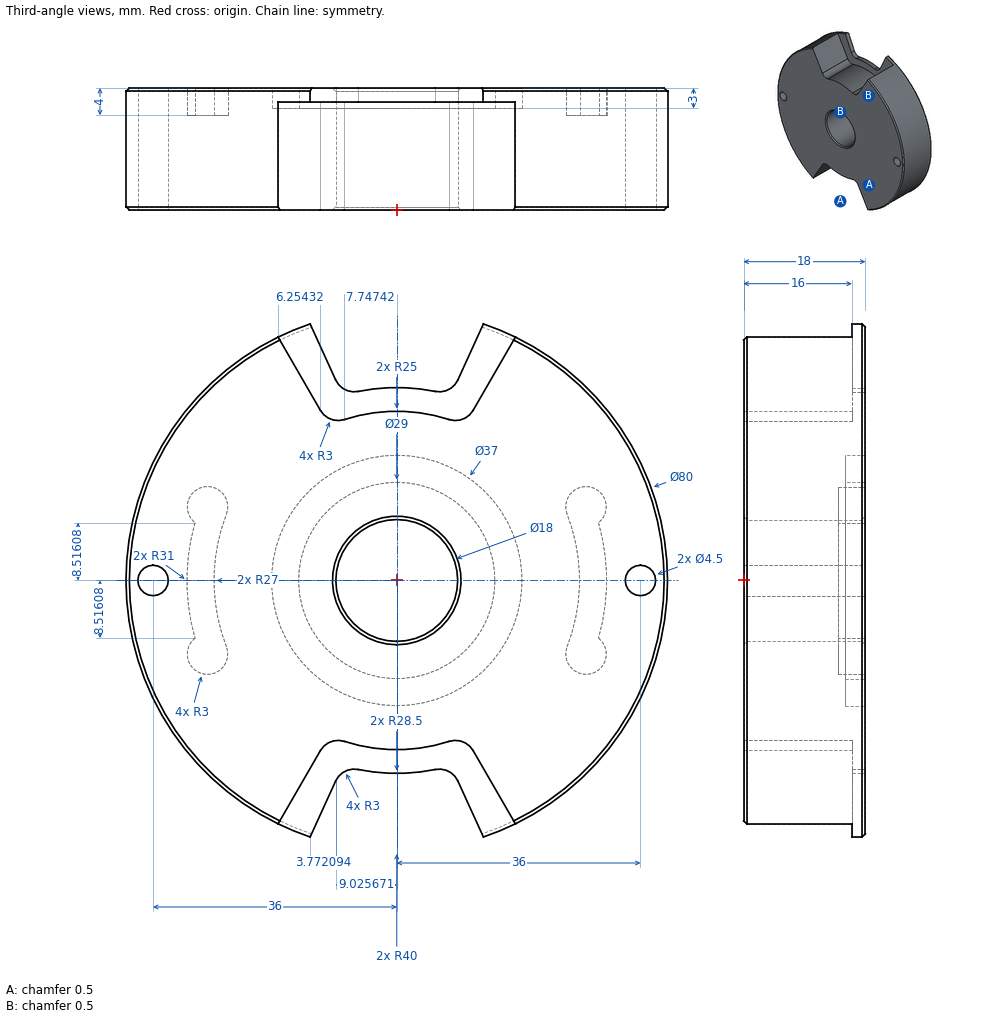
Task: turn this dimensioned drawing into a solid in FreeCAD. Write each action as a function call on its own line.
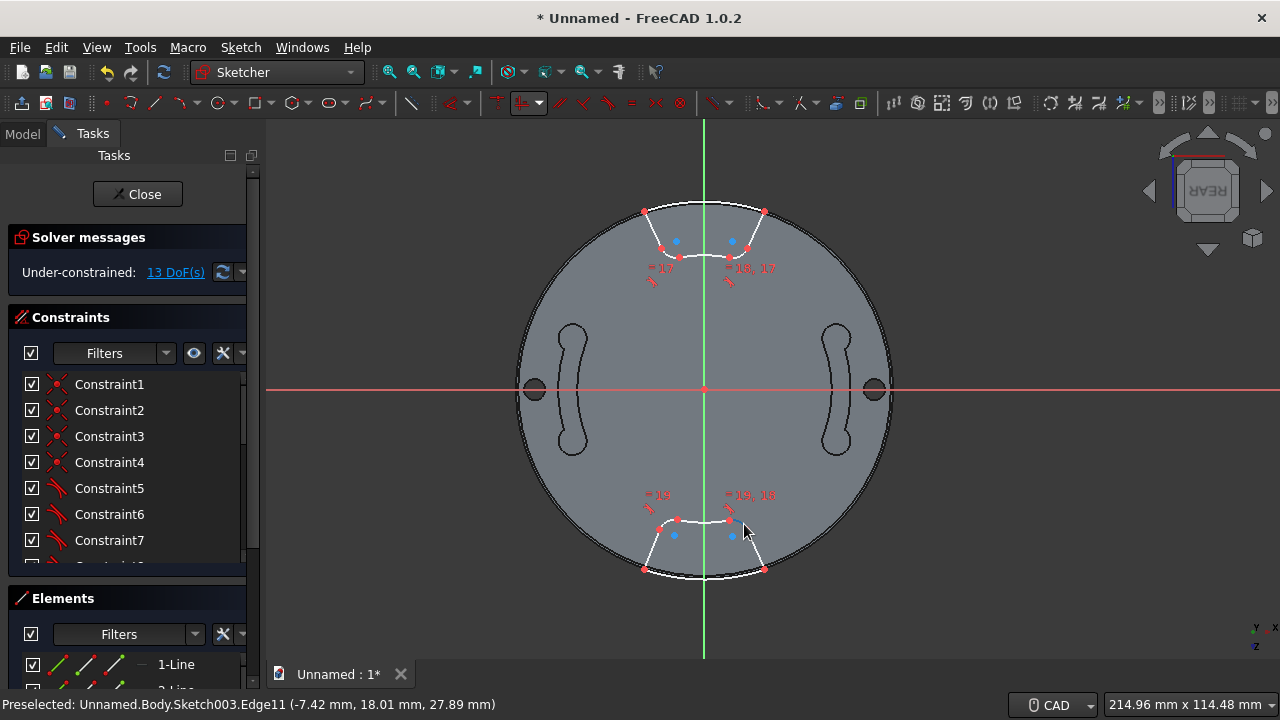
scroll(715, 256, up, 2)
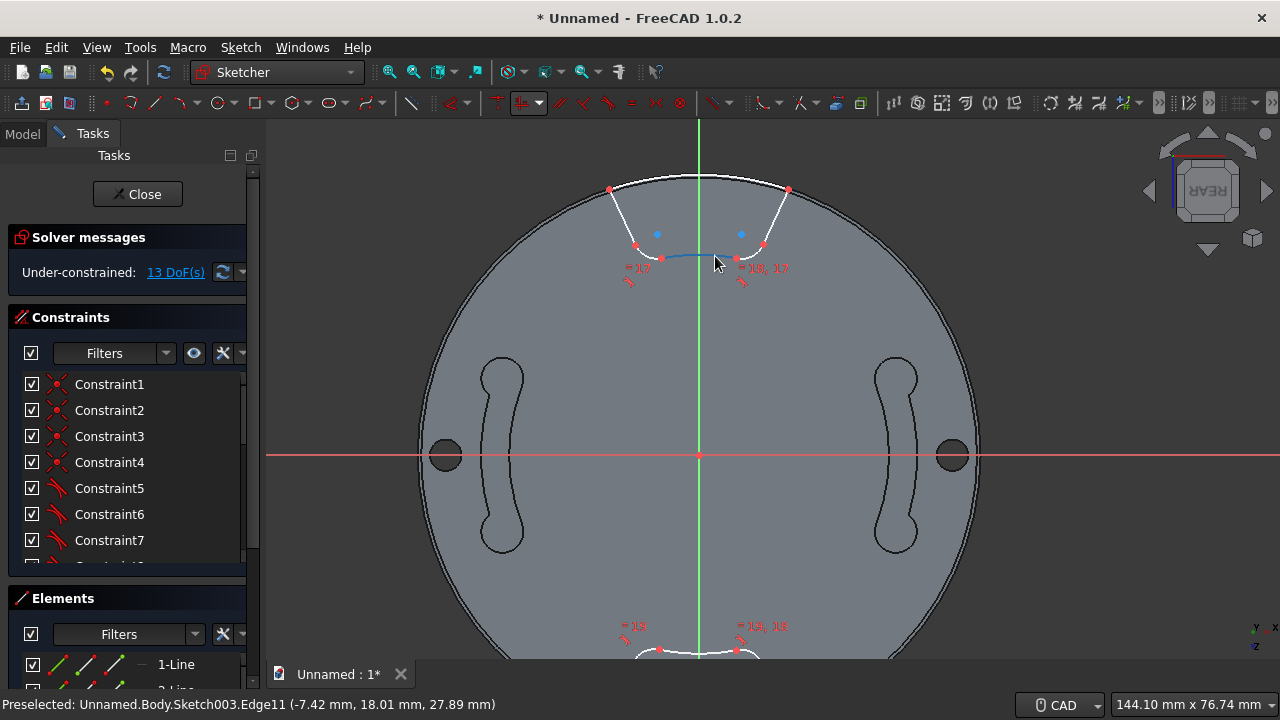
click(714, 255)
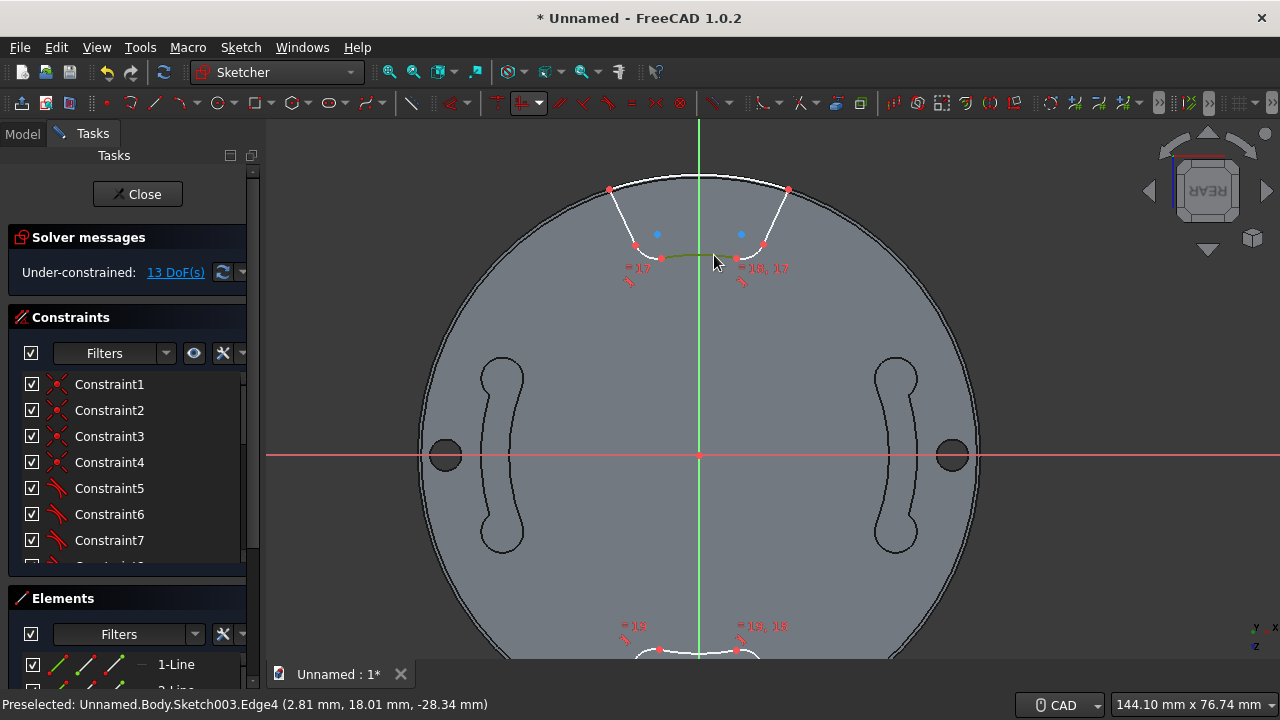
scroll(715, 254, down, 2)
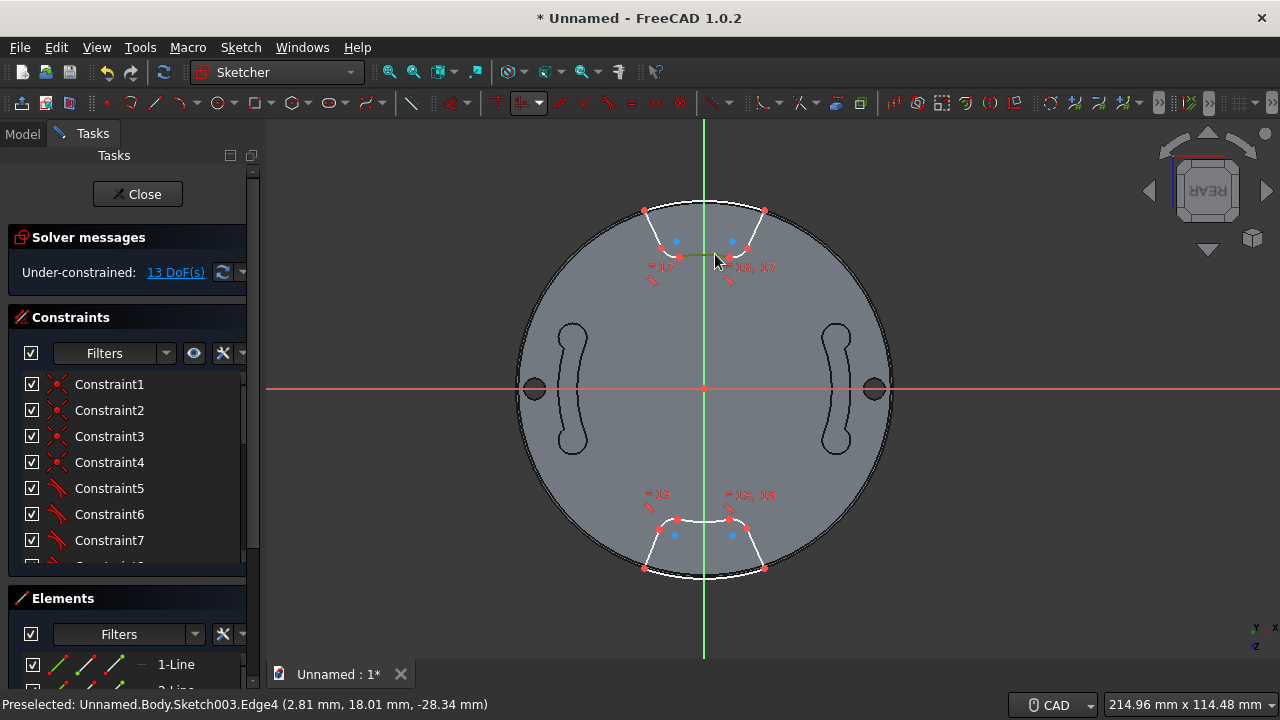
scroll(693, 522, up, 2)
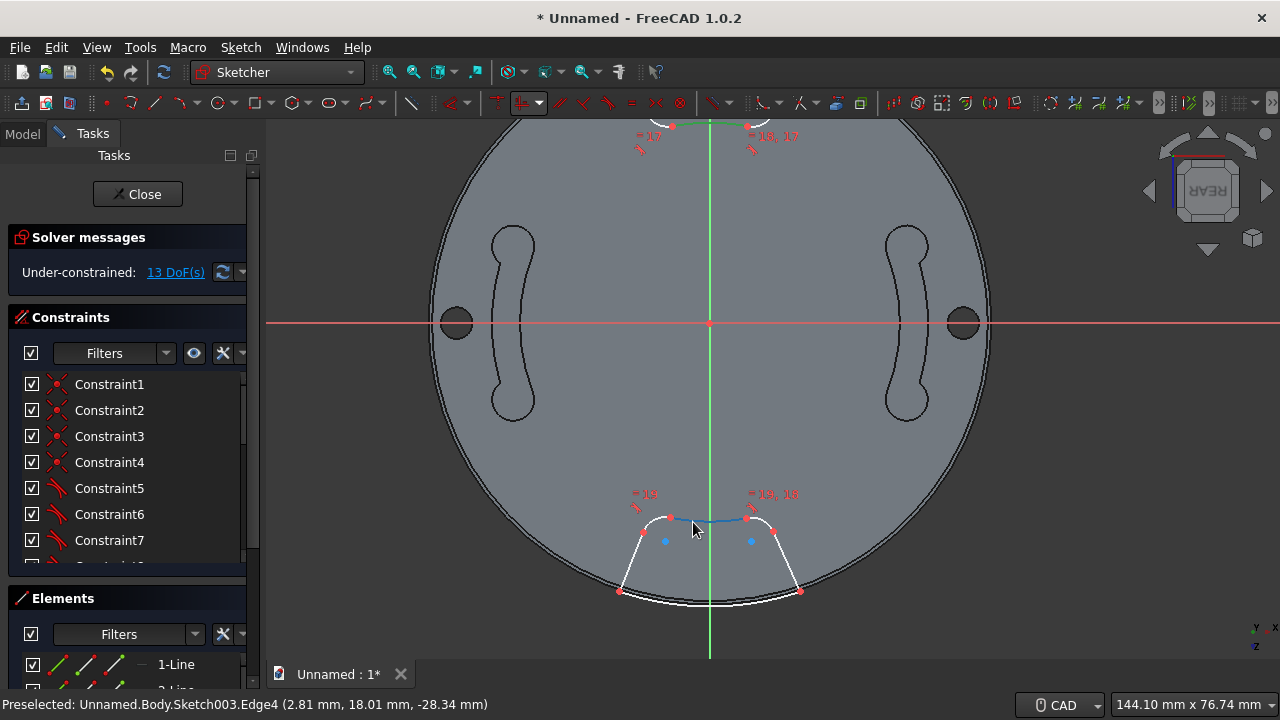
click(693, 521)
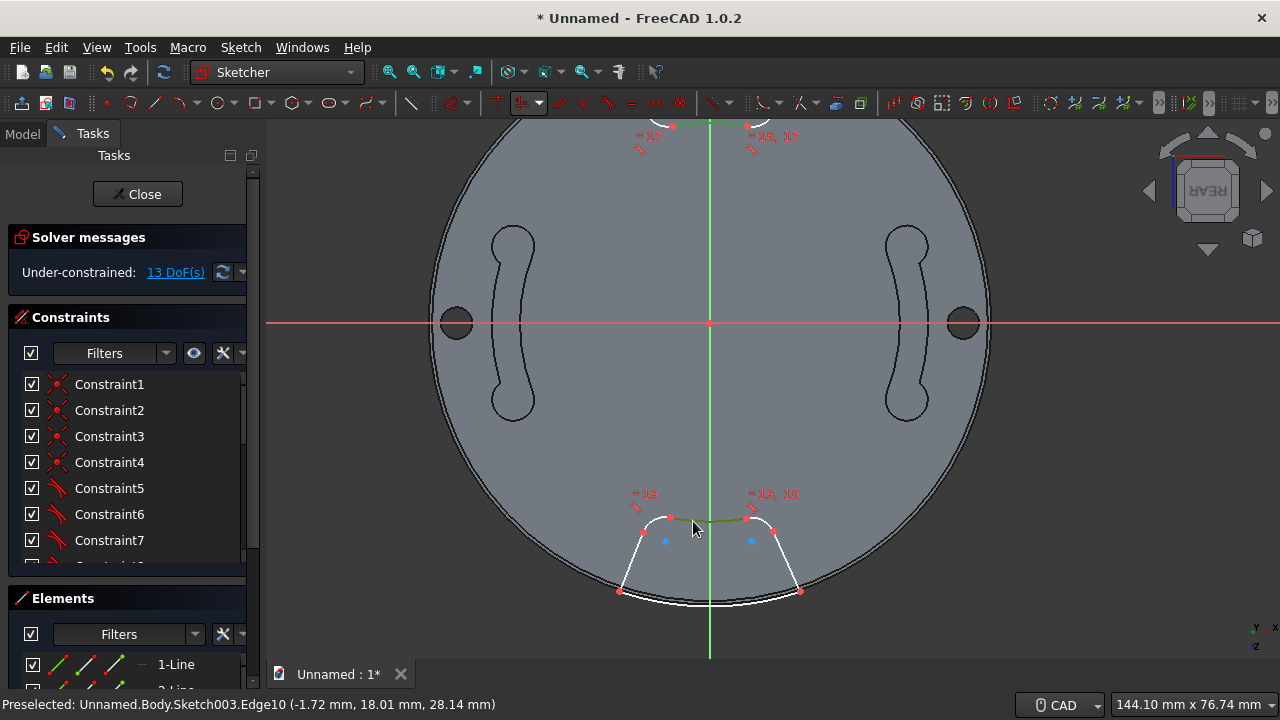
click(632, 104)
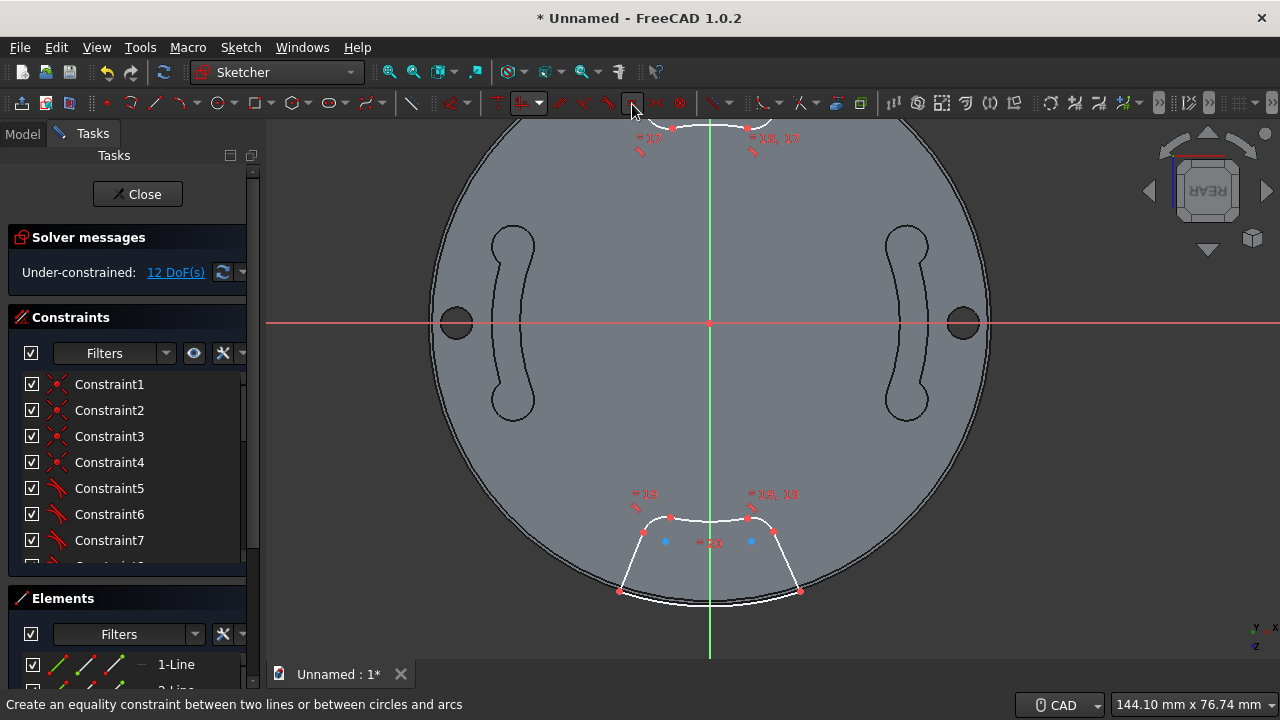
scroll(693, 523, down, 2)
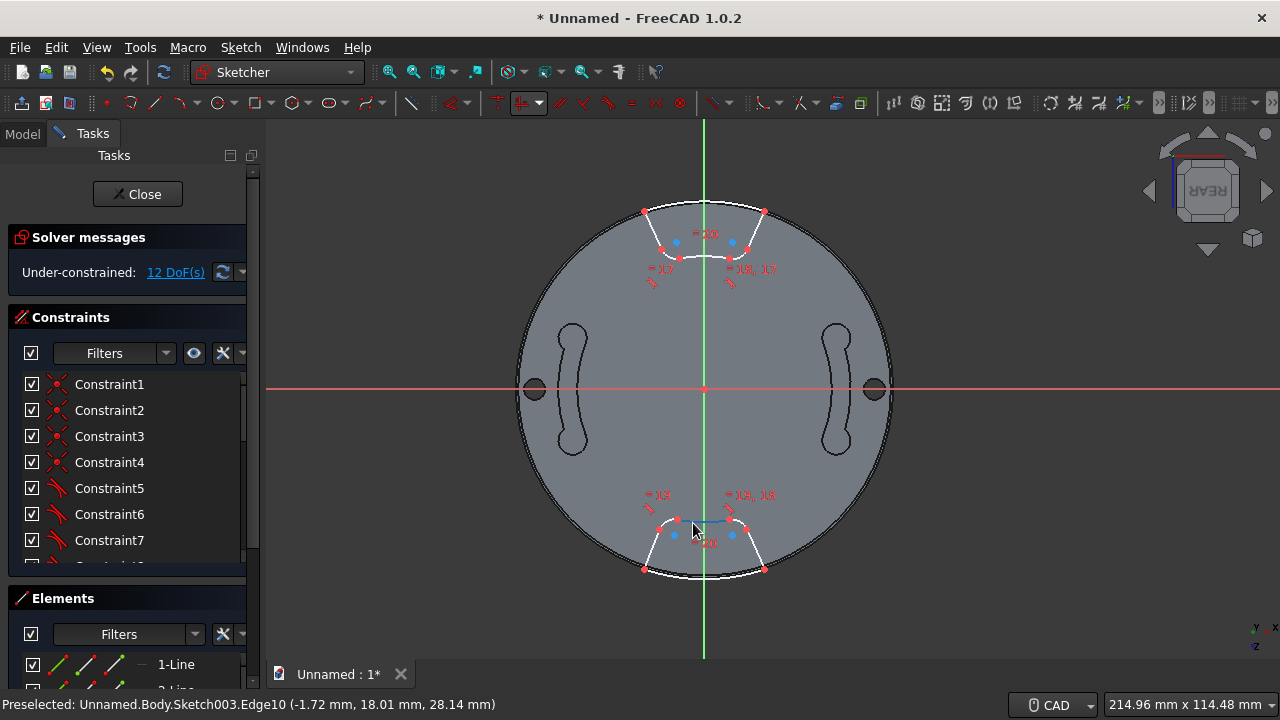
click(729, 203)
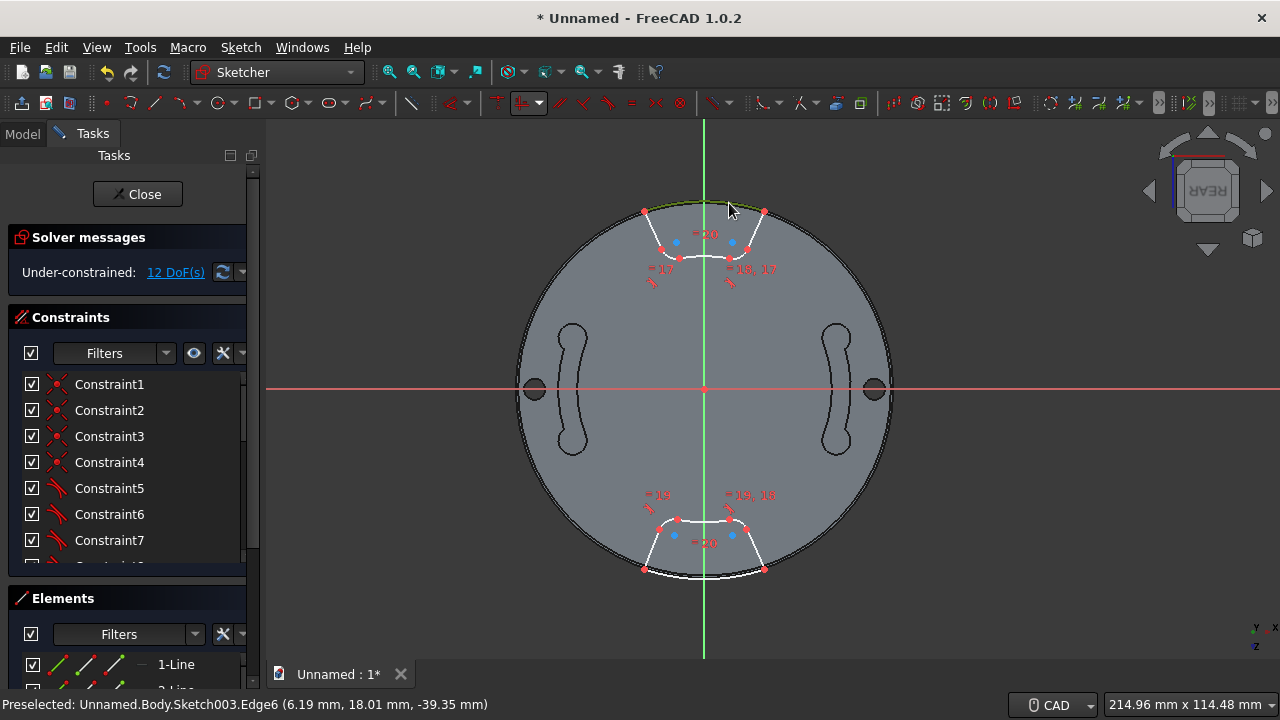
click(680, 578)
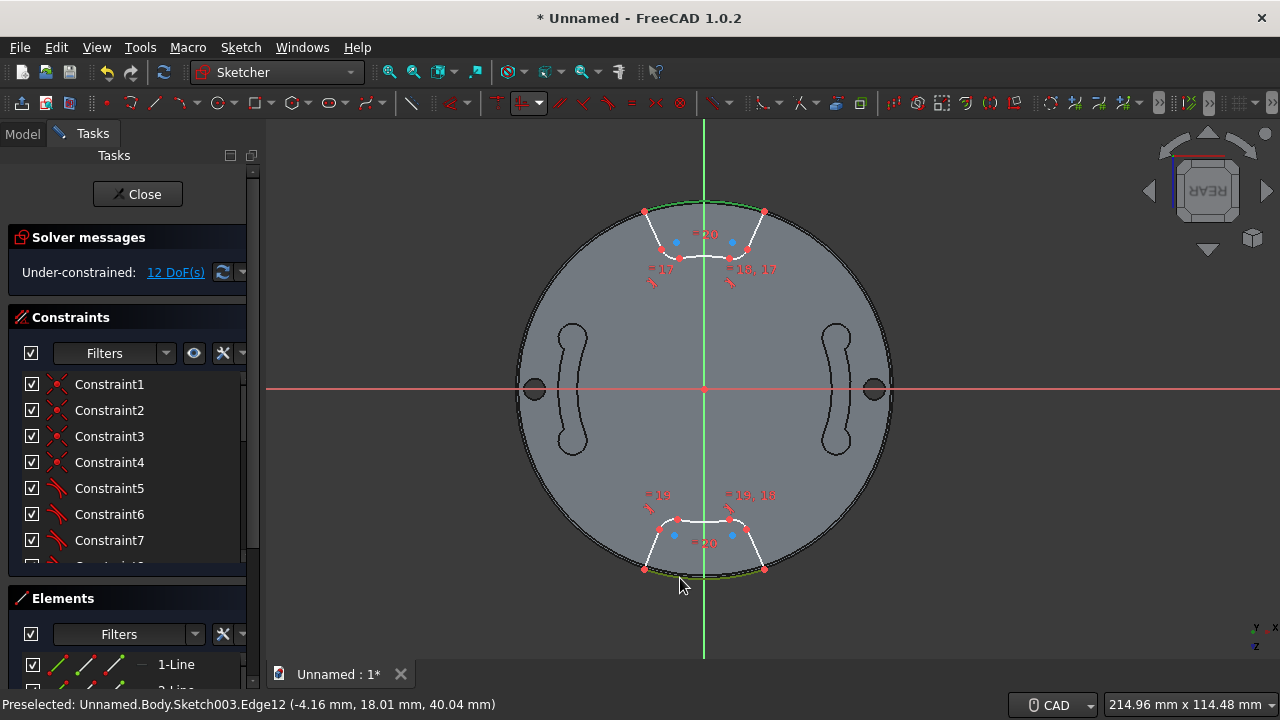
click(632, 104)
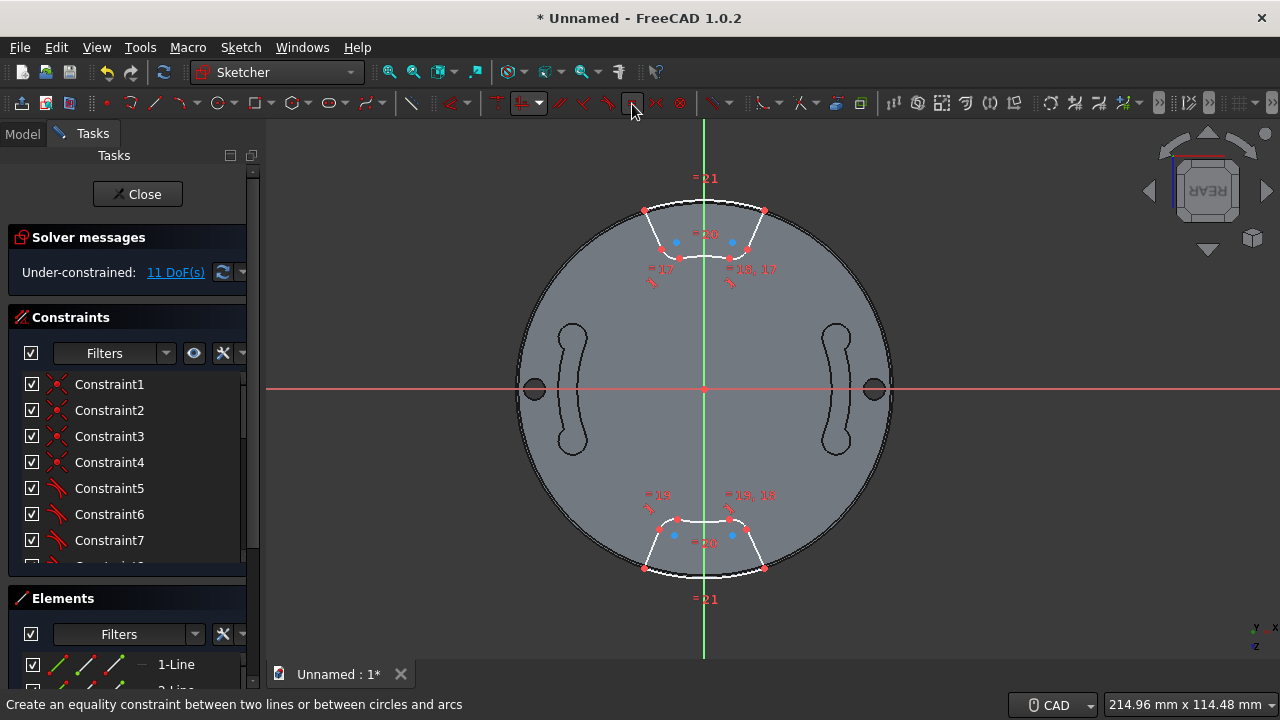
click(662, 249)